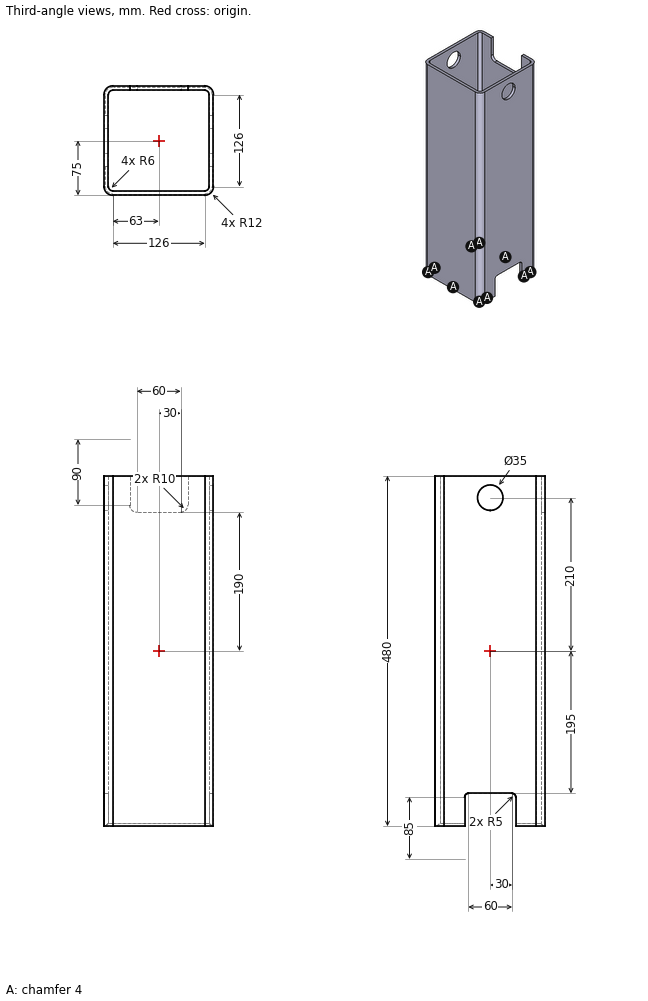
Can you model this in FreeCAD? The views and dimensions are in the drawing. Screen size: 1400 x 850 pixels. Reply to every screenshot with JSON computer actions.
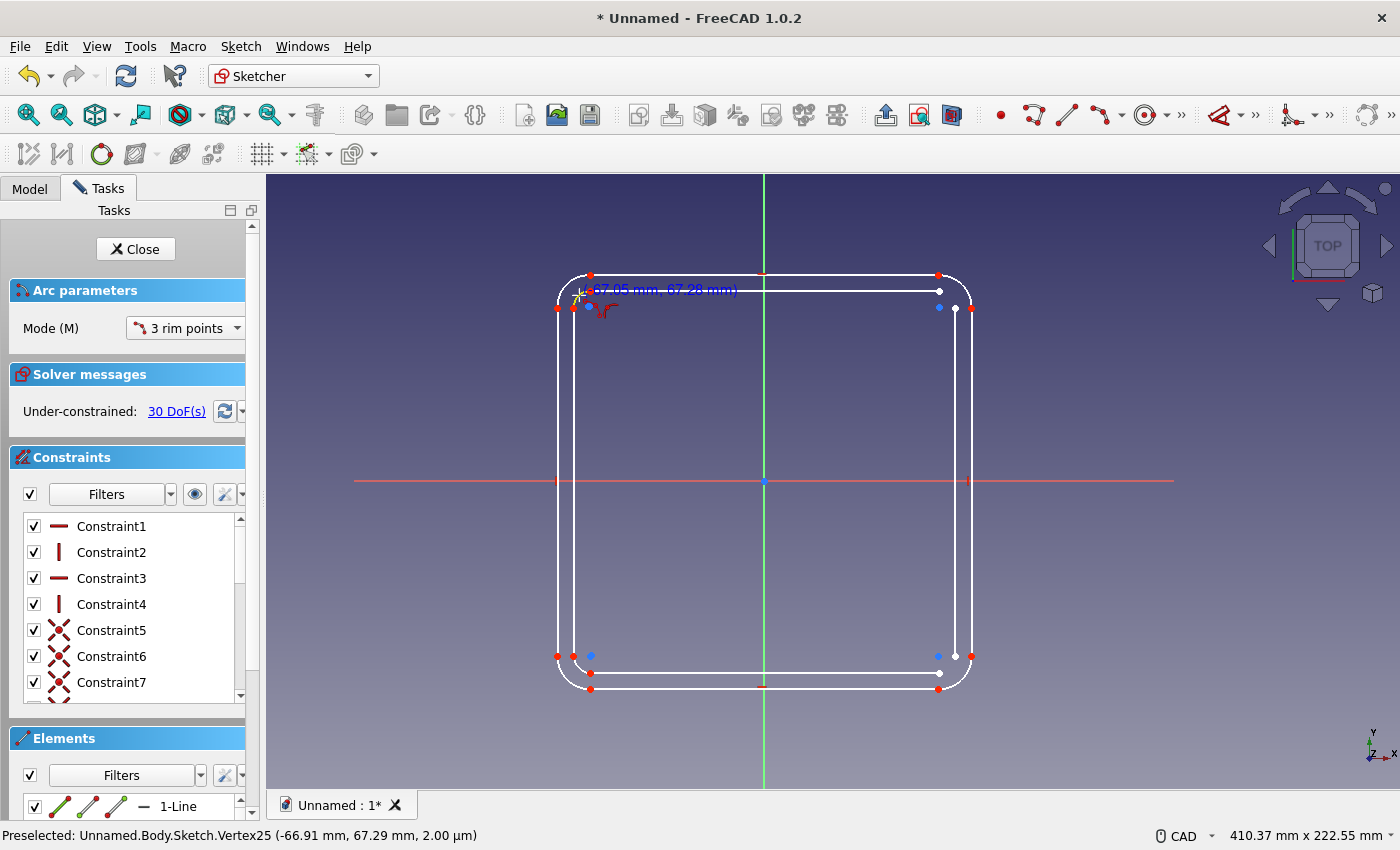
{"action": "left_click", "coordinate": [939, 291]}
{"action": "left_click", "coordinate": [955, 308]}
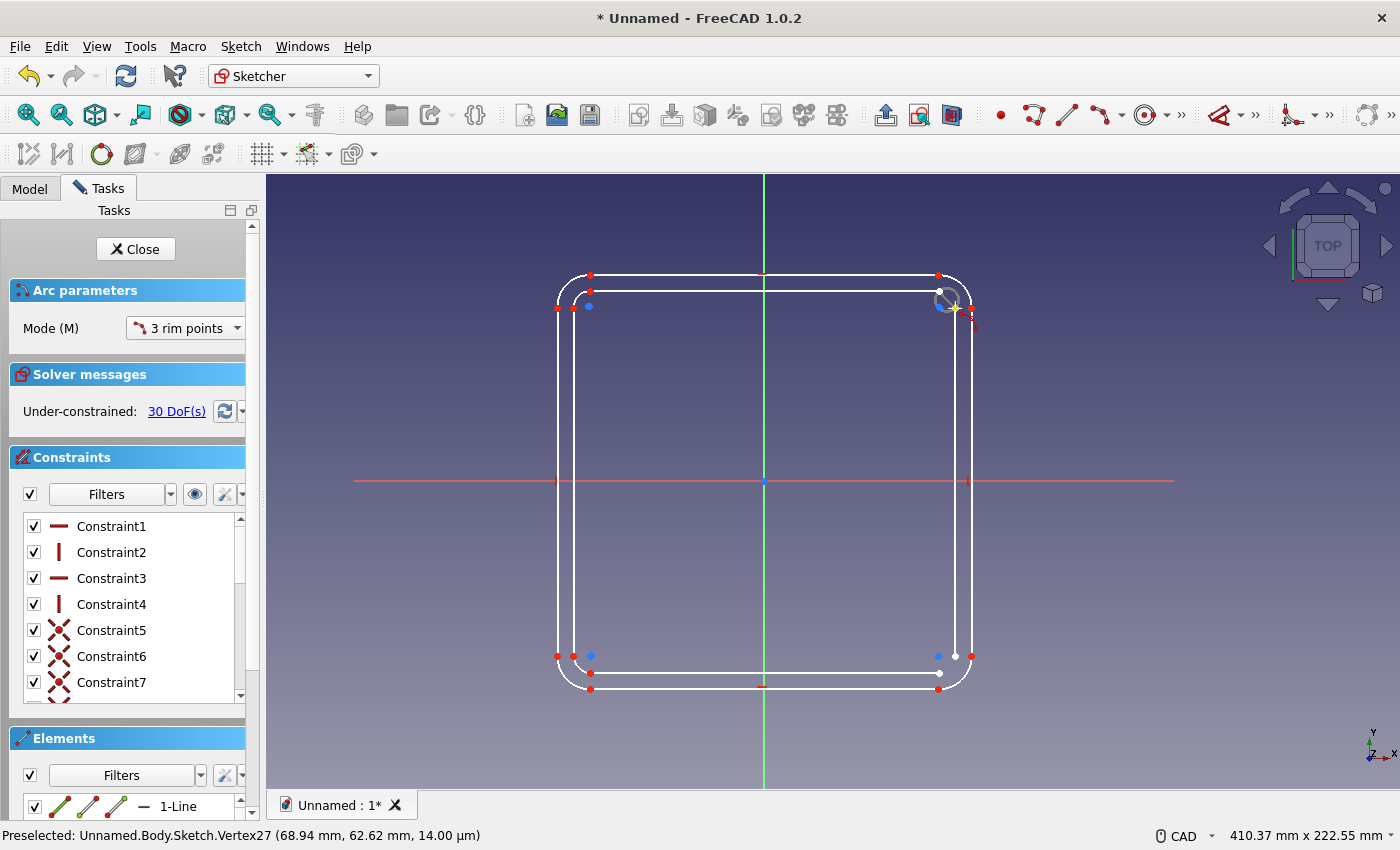
{"action": "scroll", "coordinate": [950, 296], "scroll_direction": "up", "scroll_amount": 6}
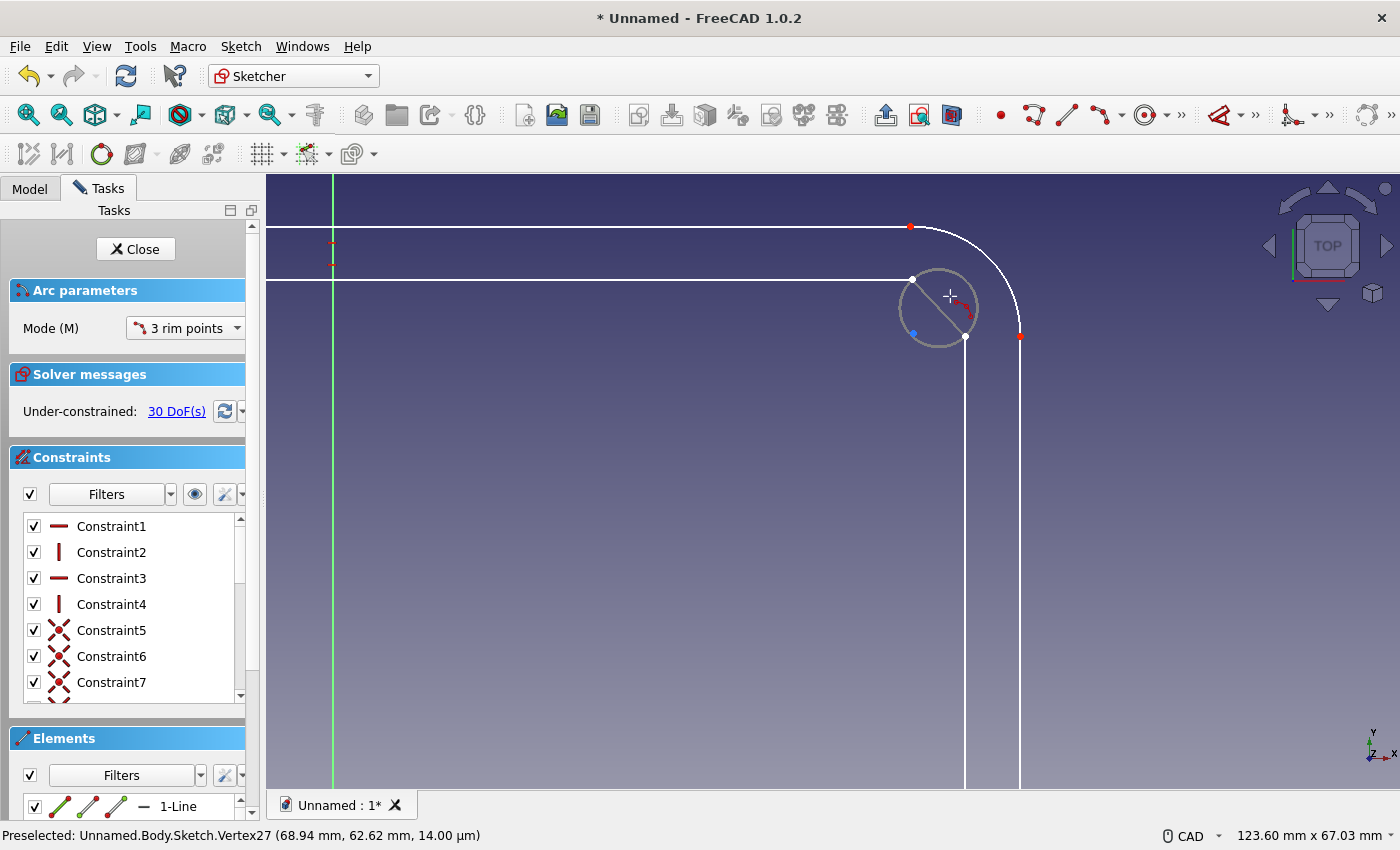
{"action": "left_click", "coordinate": [950, 294]}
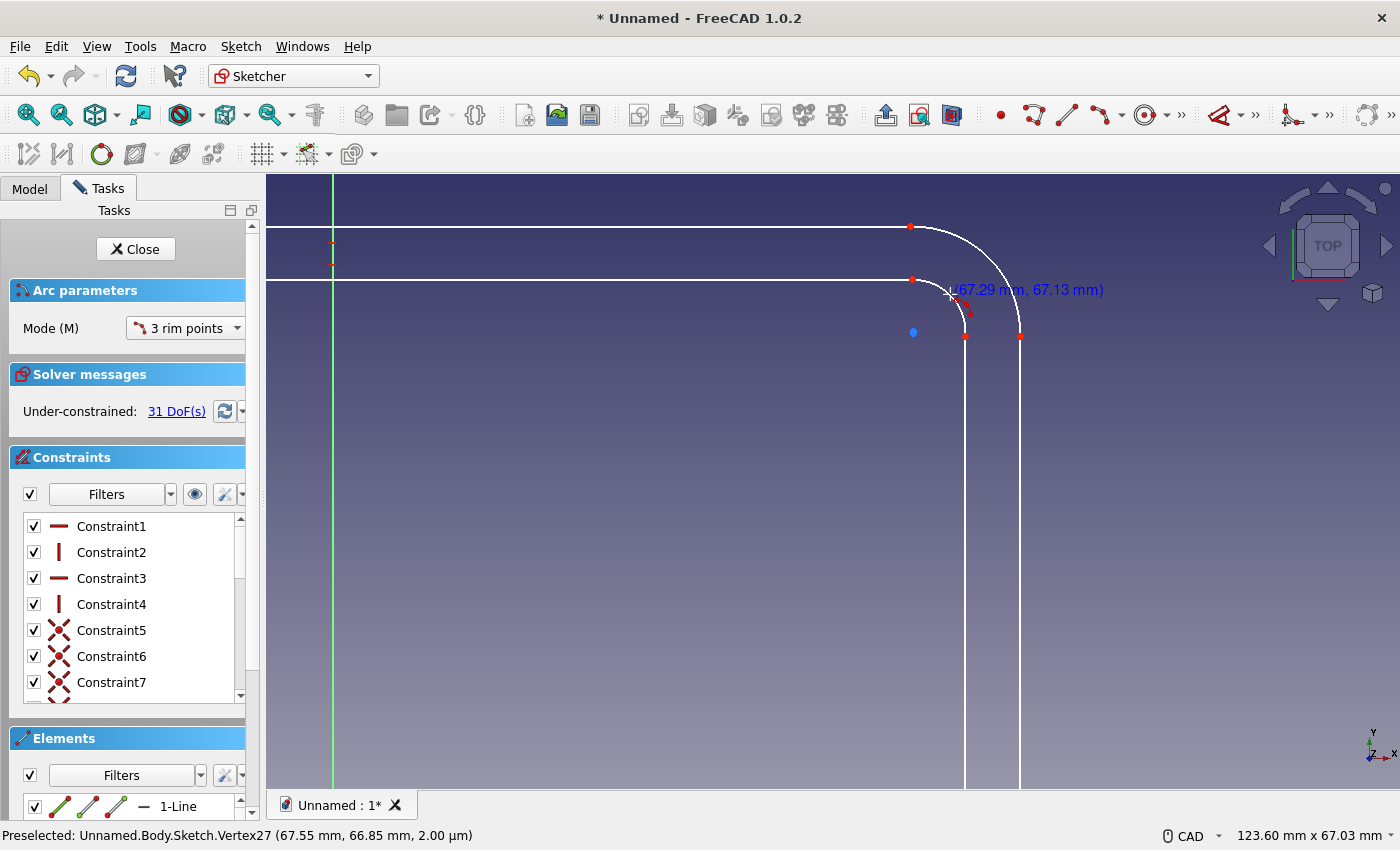
{"action": "scroll", "coordinate": [951, 296], "scroll_direction": "down", "scroll_amount": 6}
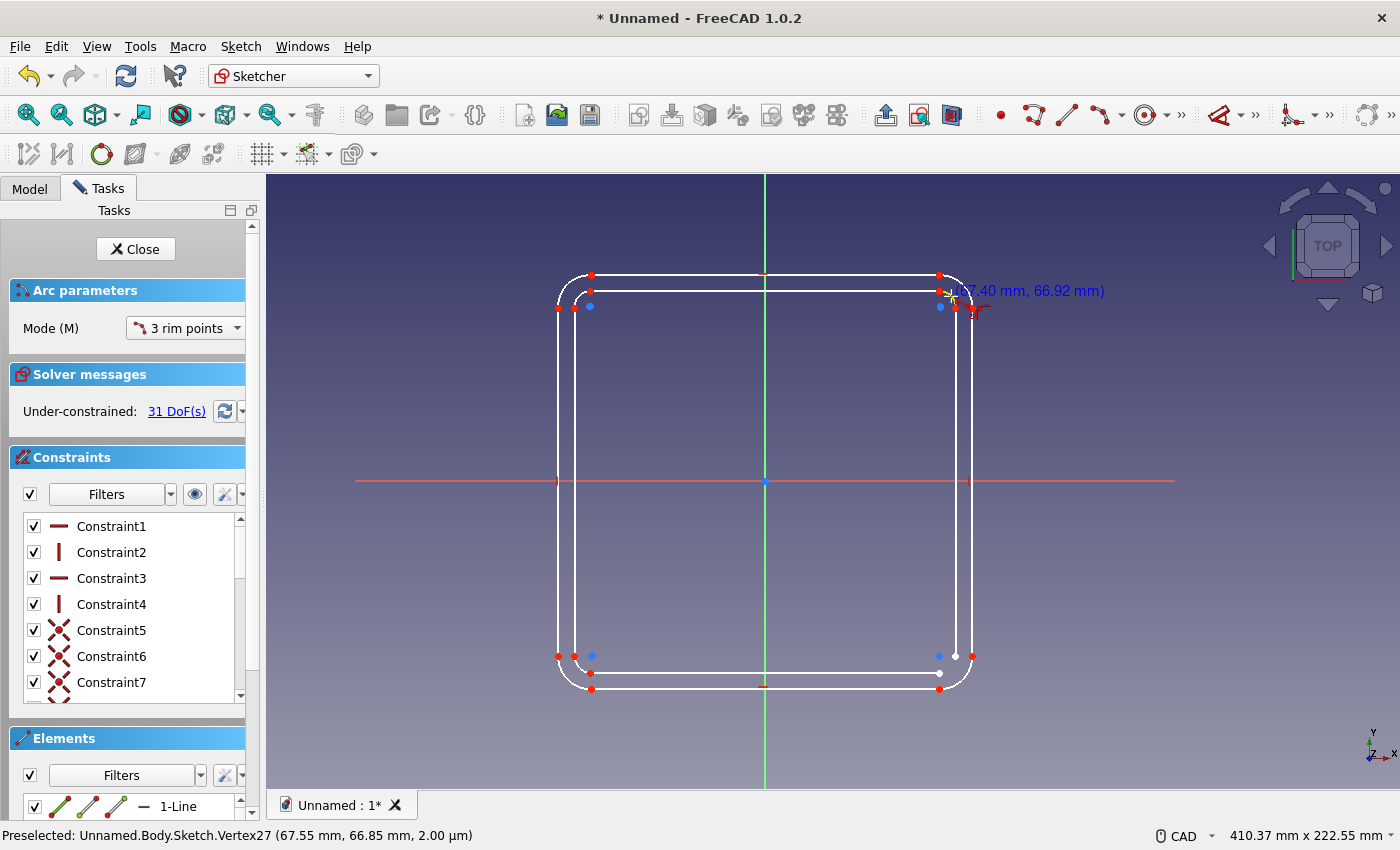
{"action": "left_click", "coordinate": [956, 656]}
{"action": "left_click", "coordinate": [940, 673]}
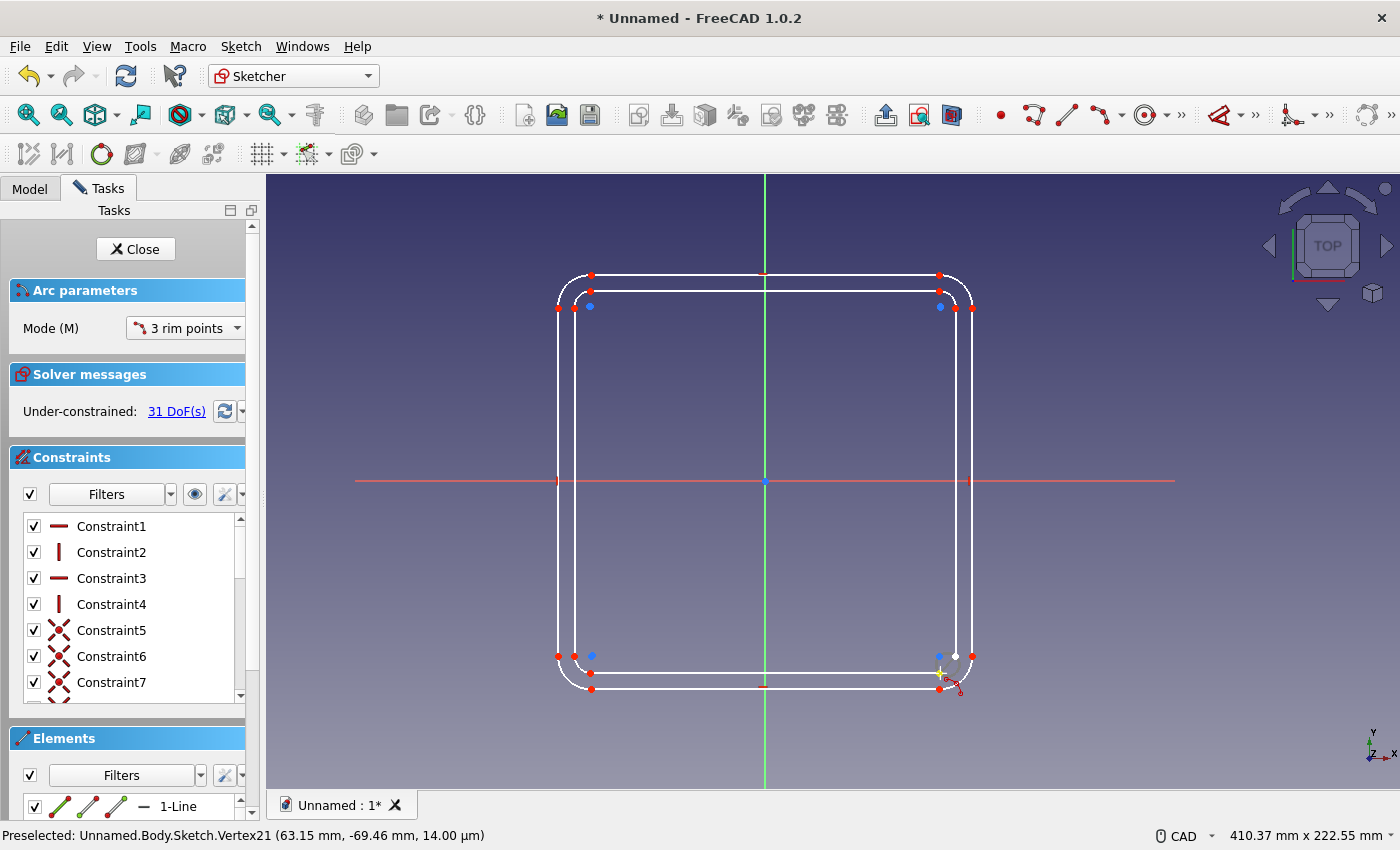
{"action": "scroll", "coordinate": [951, 667], "scroll_direction": "up", "scroll_amount": 6}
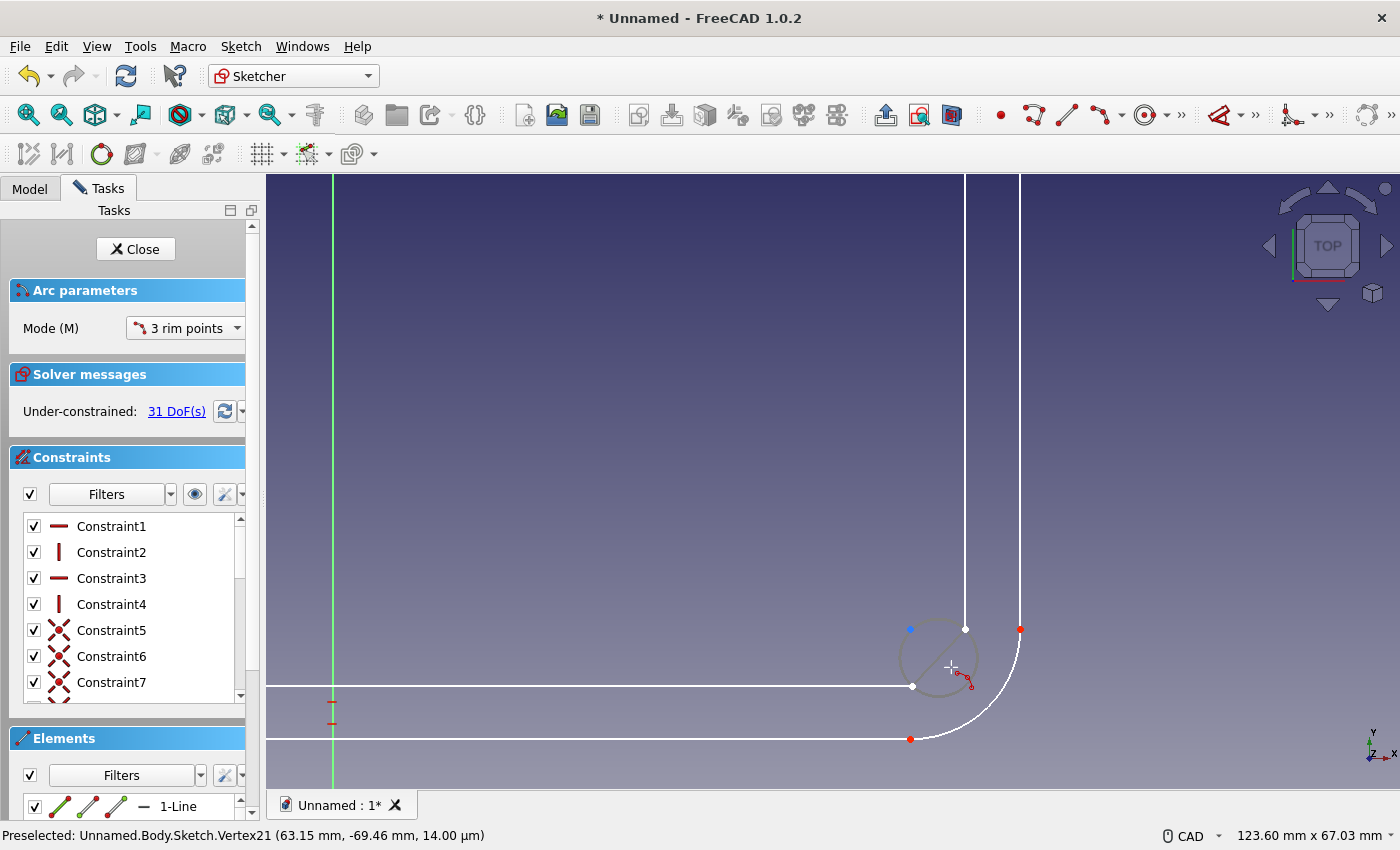
{"action": "left_click", "coordinate": [950, 666]}
{"action": "key", "text": "Escape"}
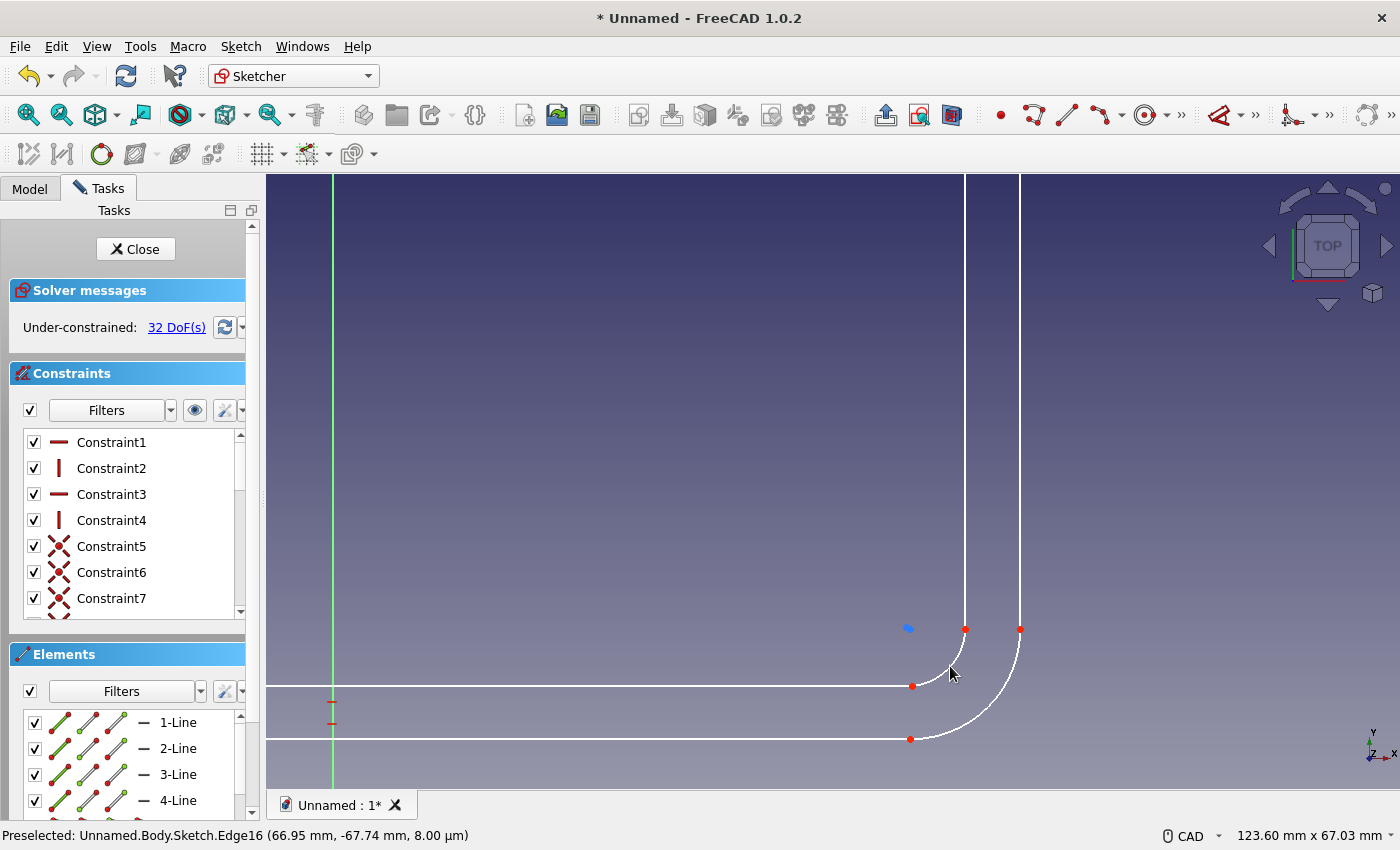
{"action": "left_click", "coordinate": [564, 739]}